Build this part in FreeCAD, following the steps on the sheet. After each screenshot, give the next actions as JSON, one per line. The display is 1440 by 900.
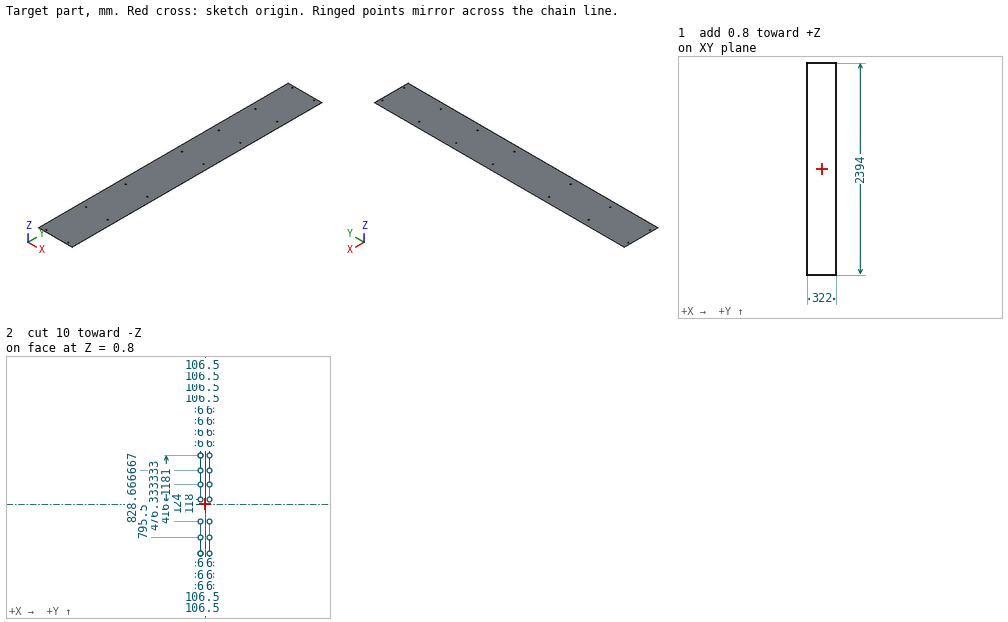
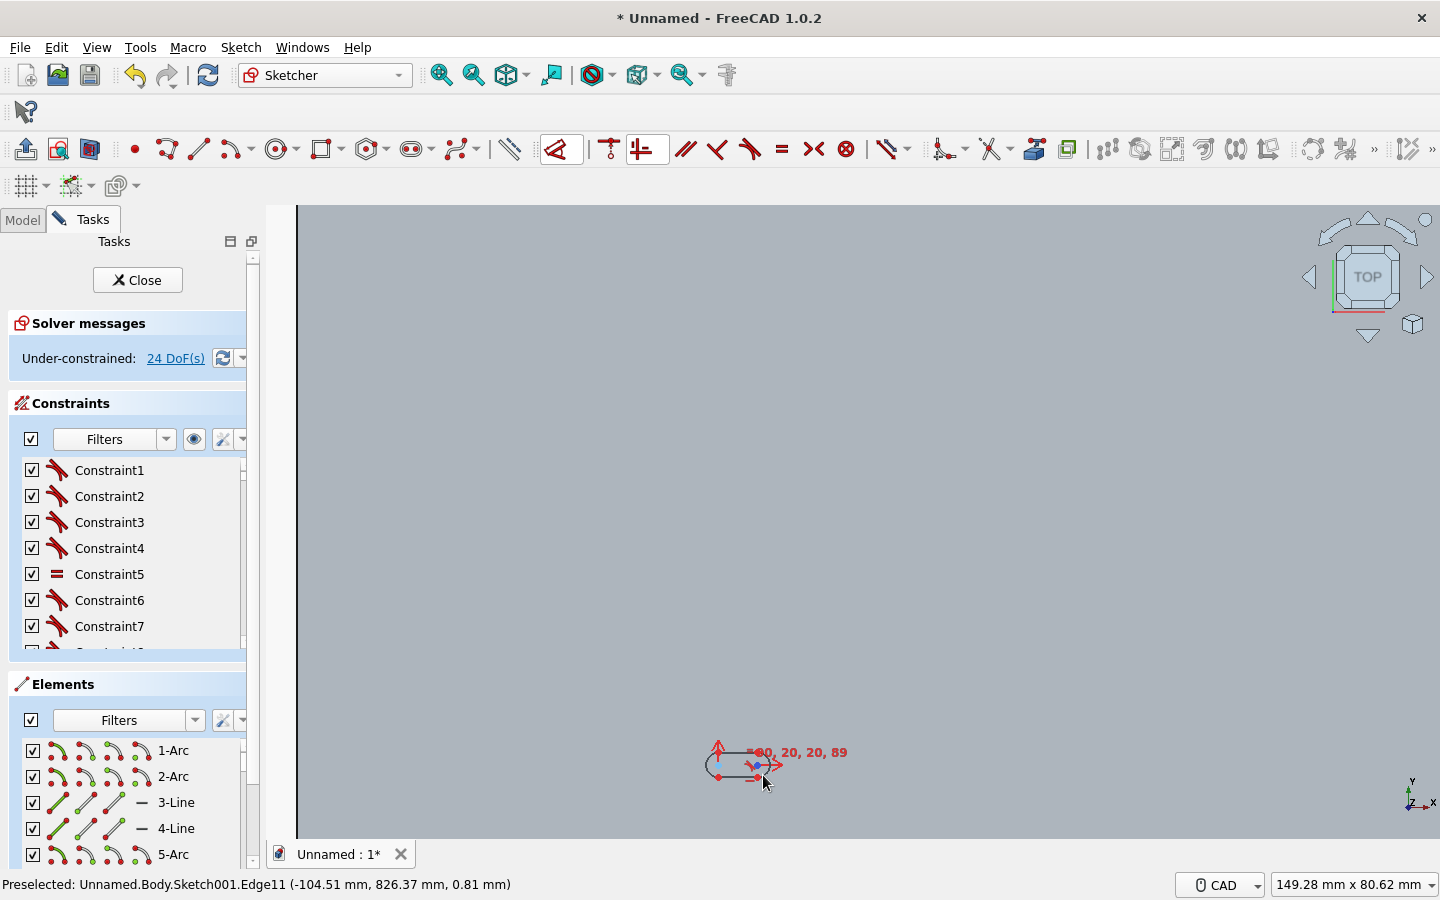
{"action": "left_click", "coordinate": [730, 753]}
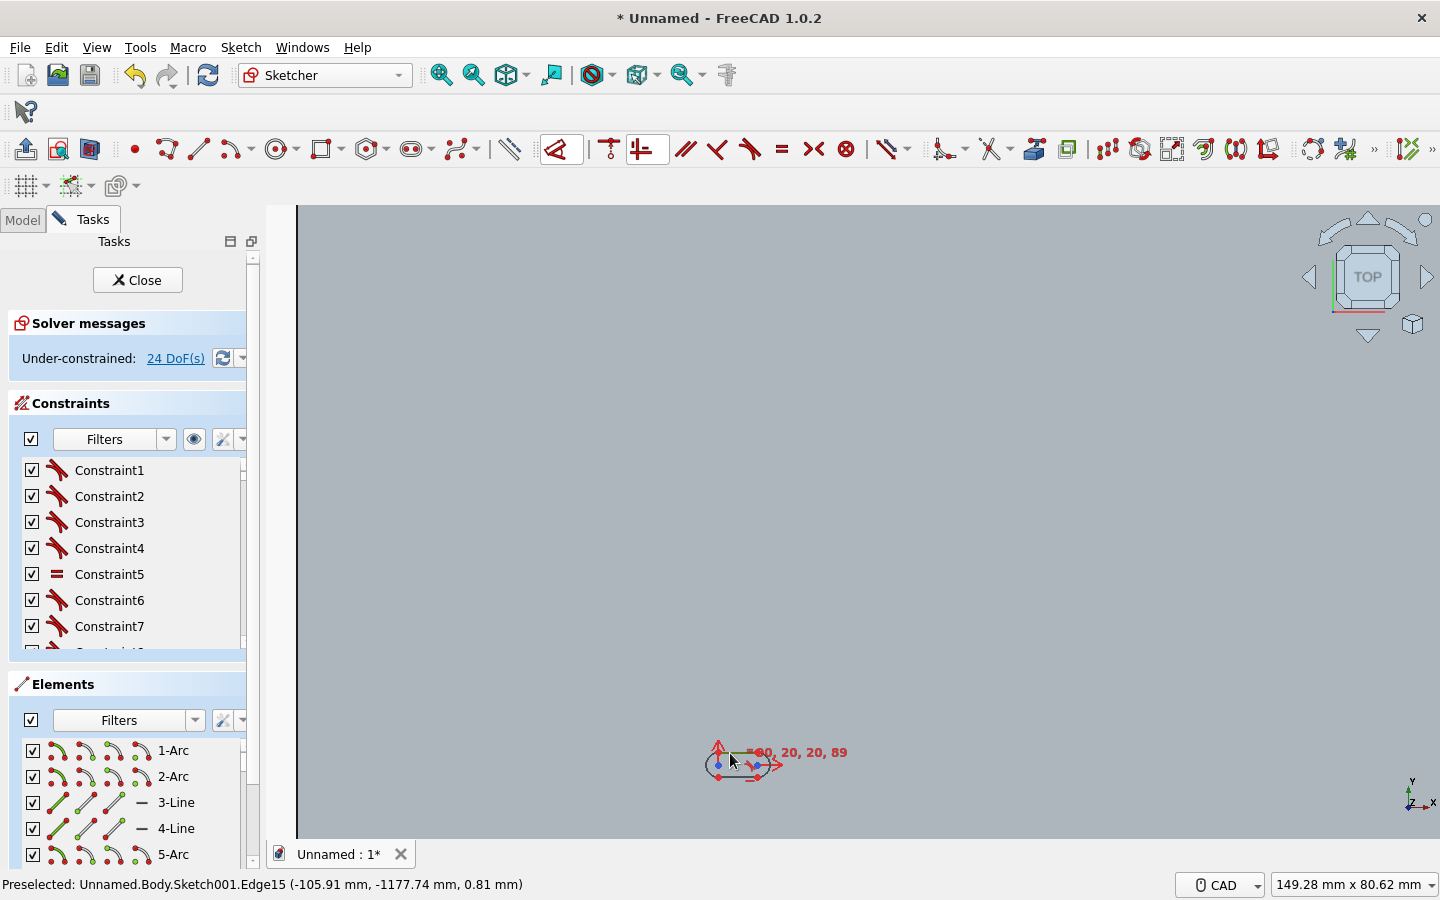
{"action": "key", "text": "l"}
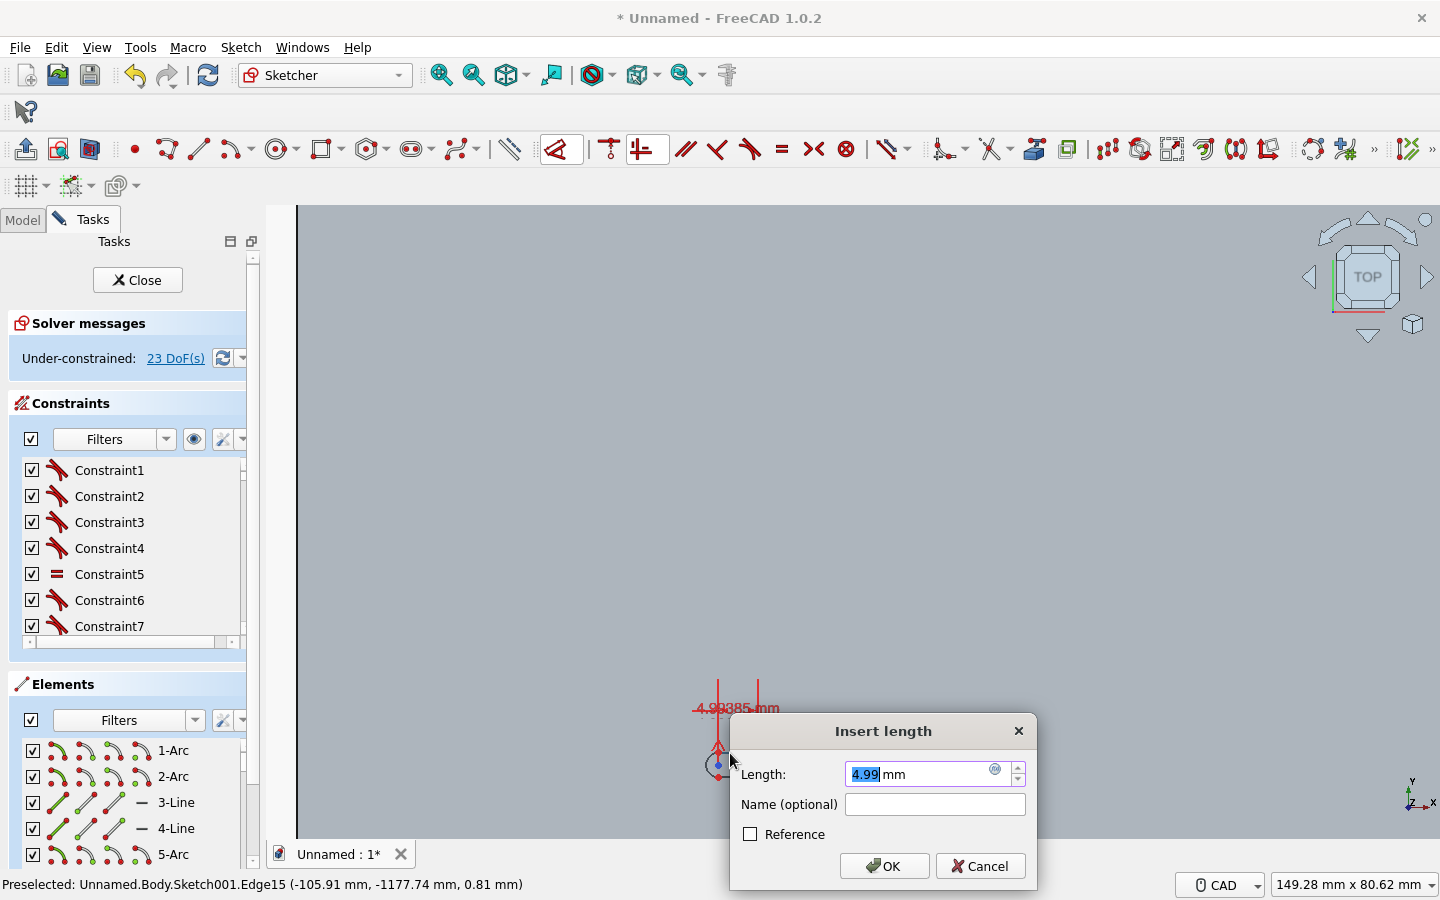
{"action": "type", "text": "6"}
{"action": "key", "text": "Return"}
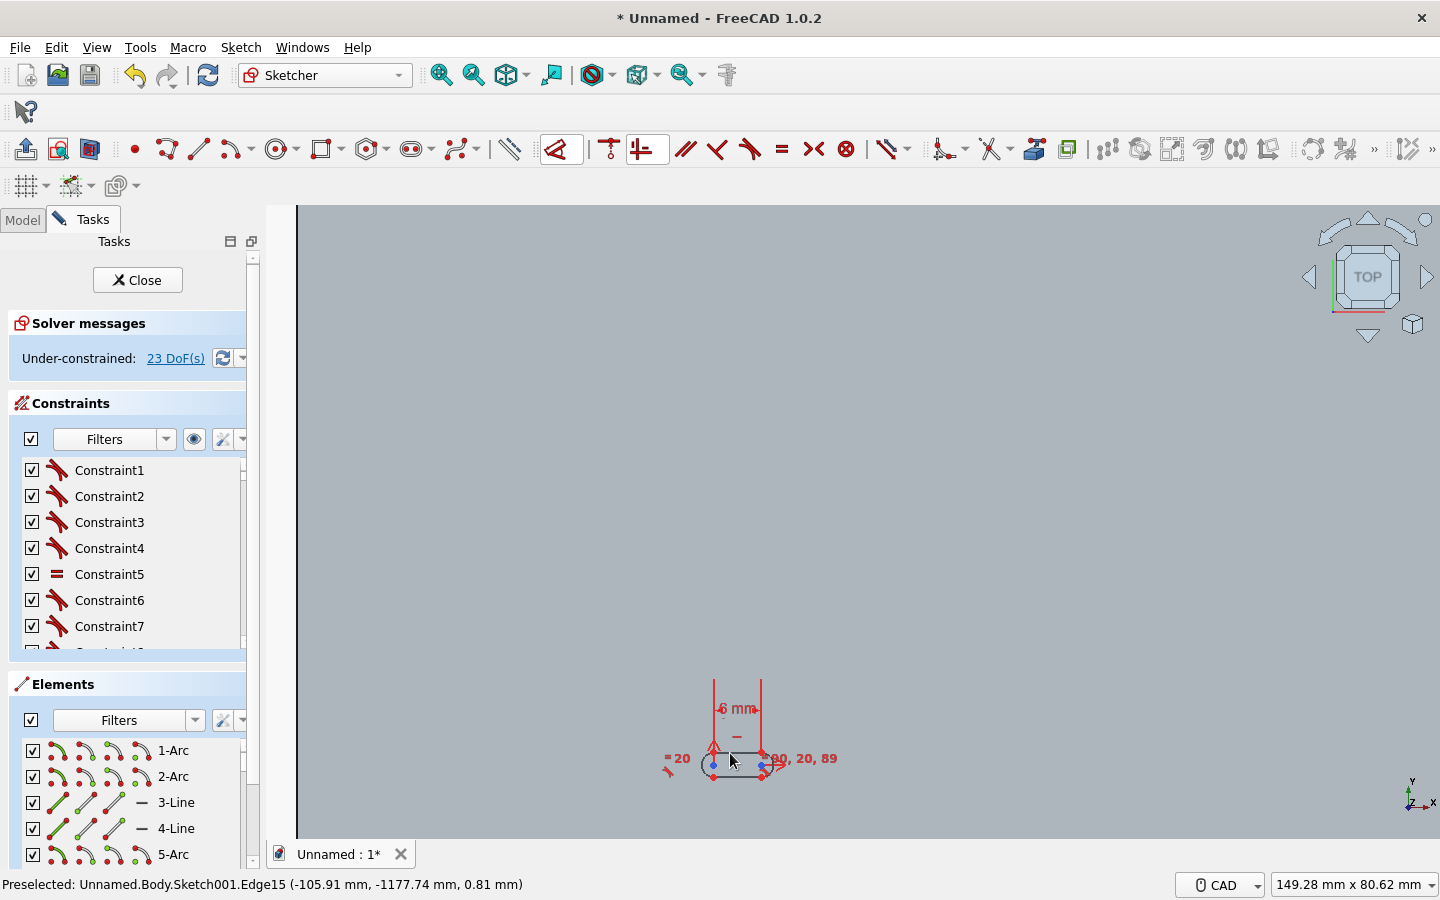
{"action": "scroll", "coordinate": [763, 776], "scroll_direction": "down", "scroll_amount": 18}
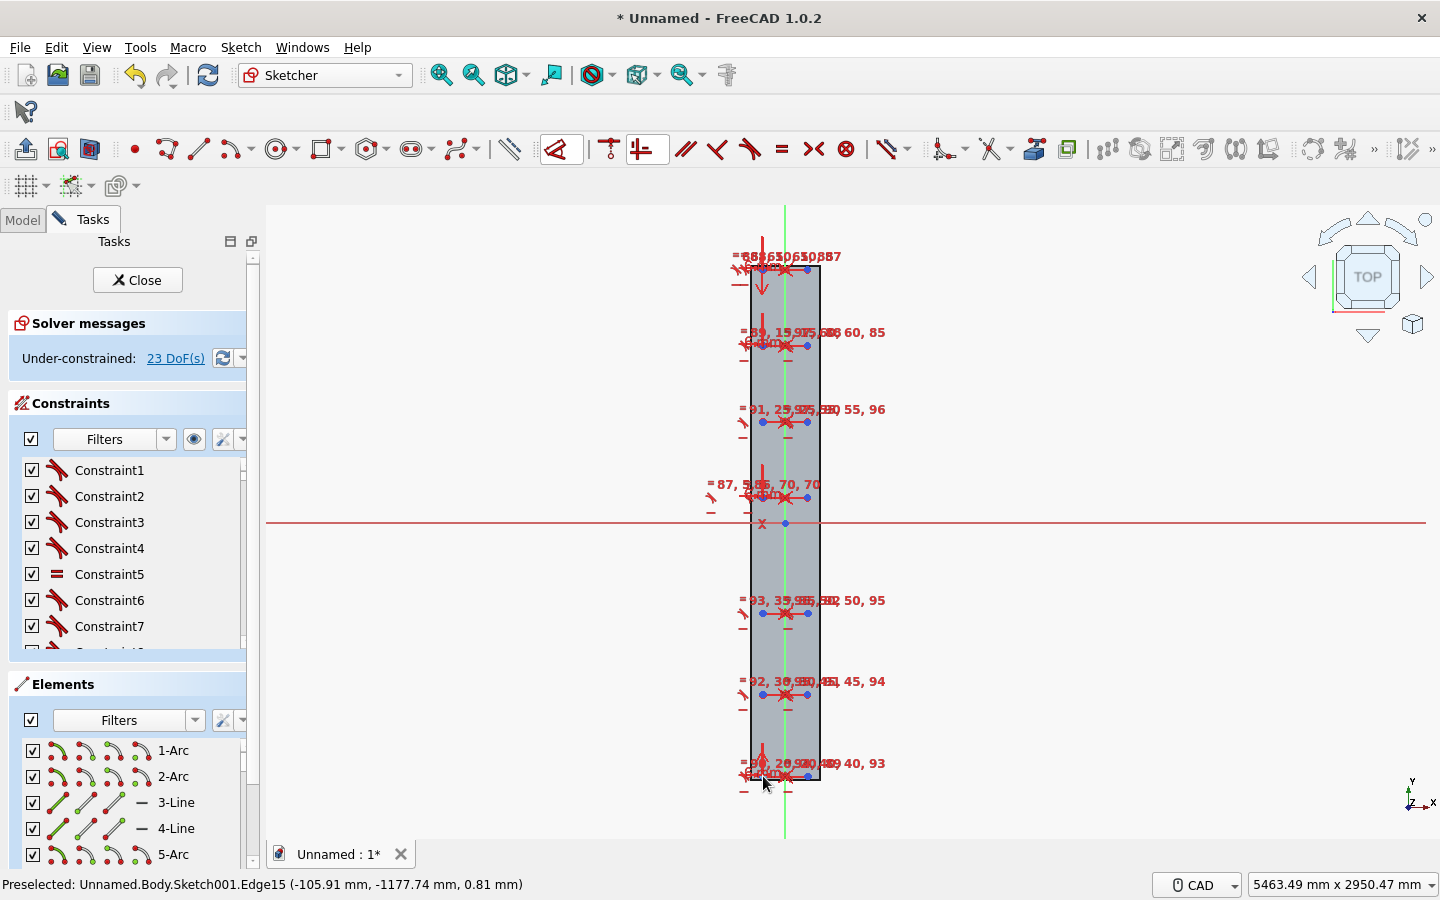
{"action": "scroll", "coordinate": [763, 422], "scroll_direction": "up", "scroll_amount": 18}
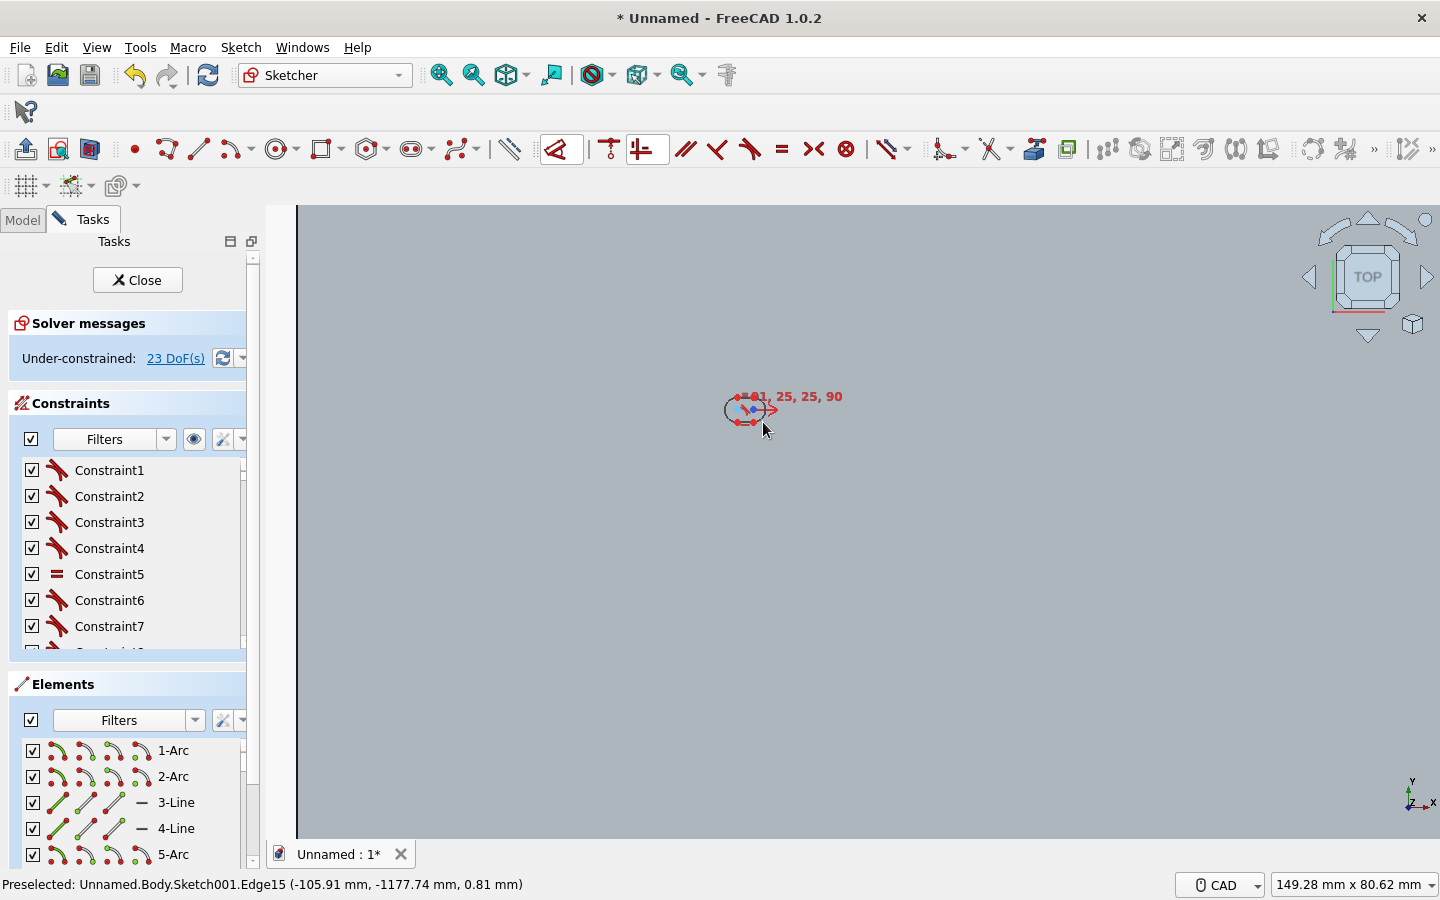
{"action": "scroll", "coordinate": [745, 398], "scroll_direction": "up", "scroll_amount": 4}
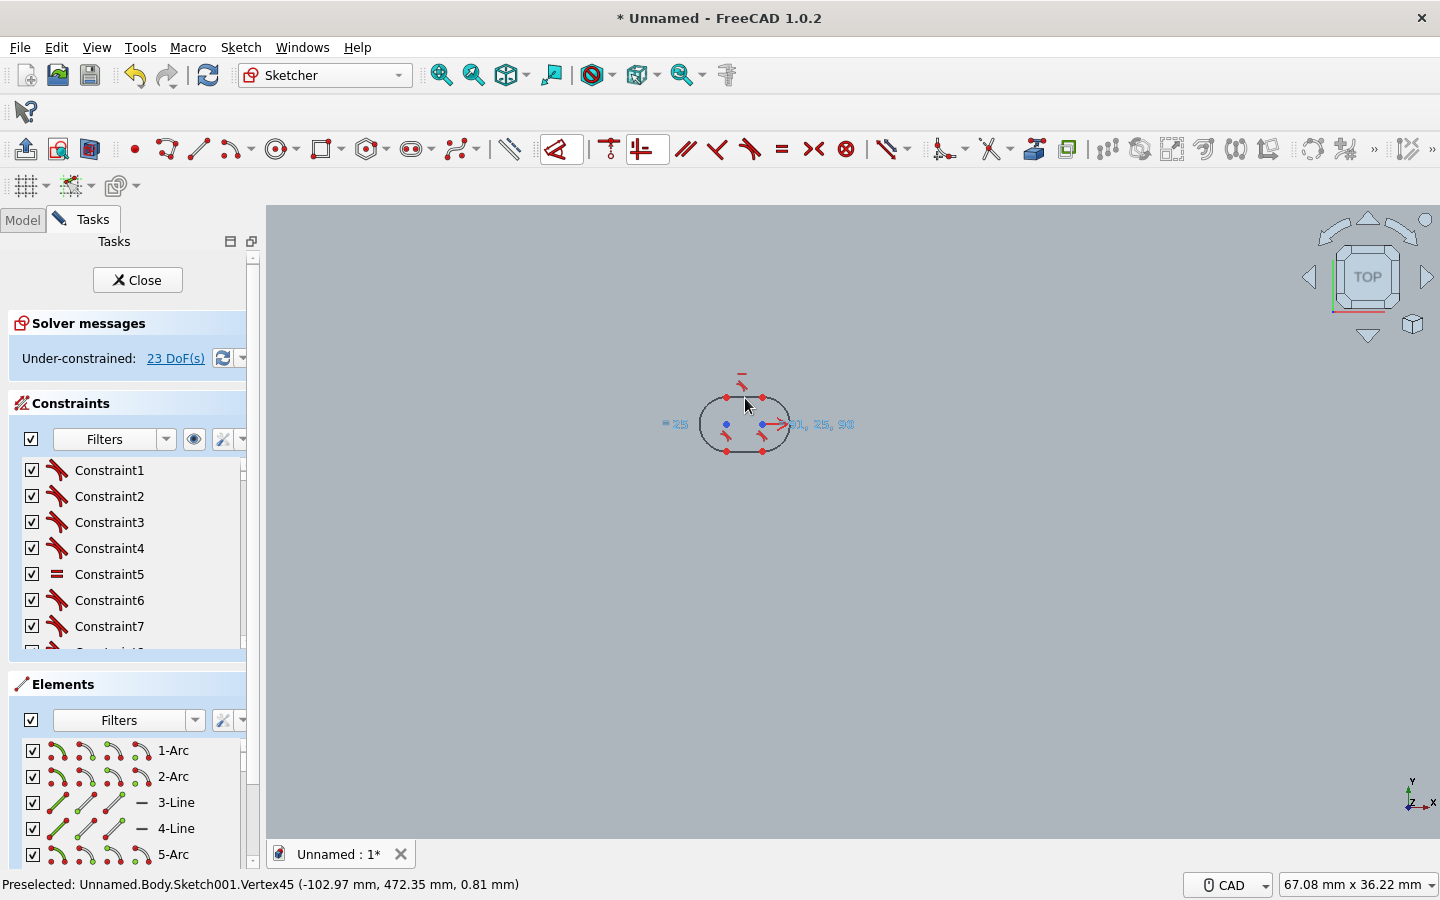
{"action": "left_click", "coordinate": [745, 397]}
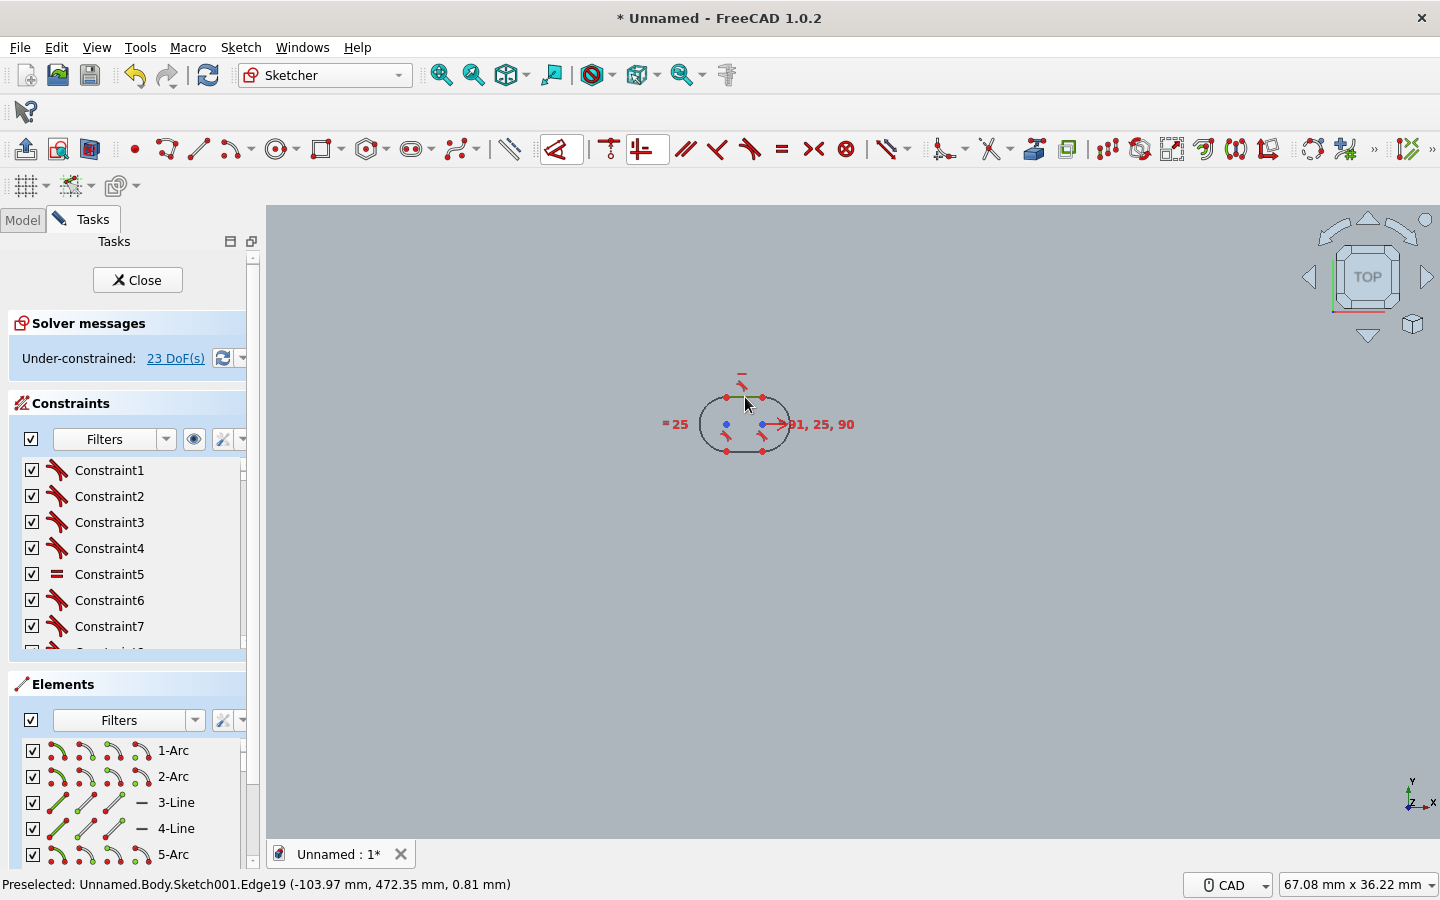
{"action": "key", "text": "l"}